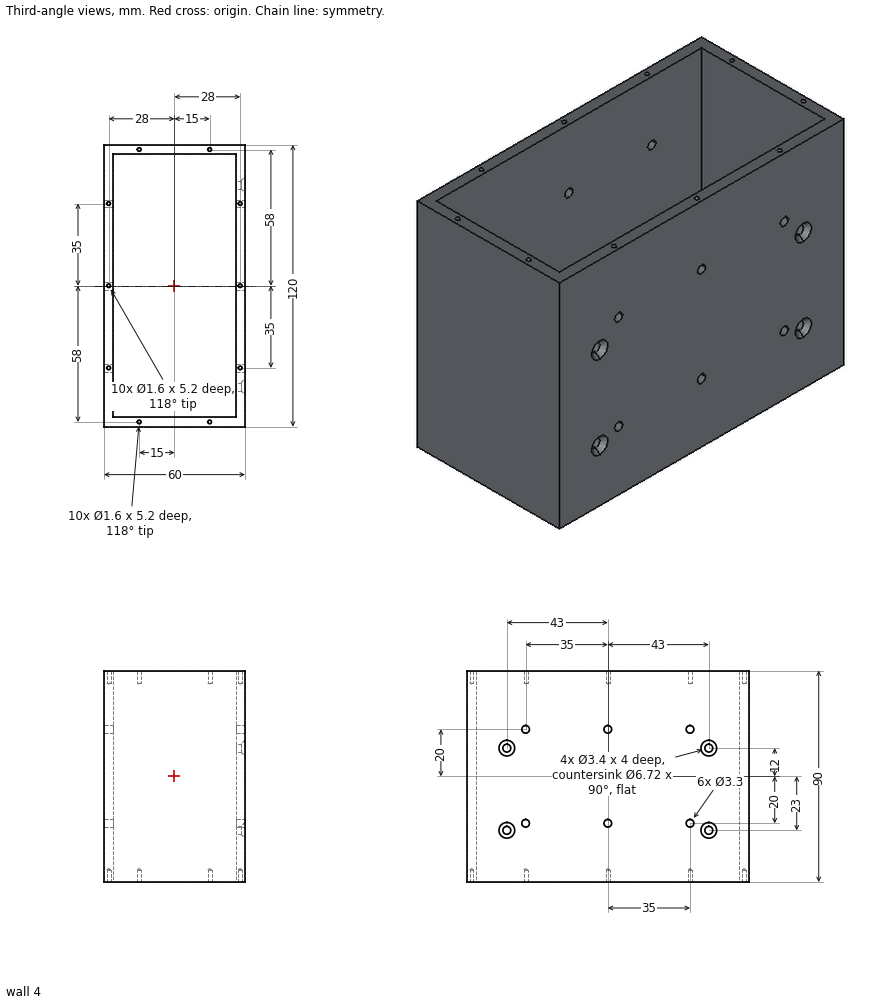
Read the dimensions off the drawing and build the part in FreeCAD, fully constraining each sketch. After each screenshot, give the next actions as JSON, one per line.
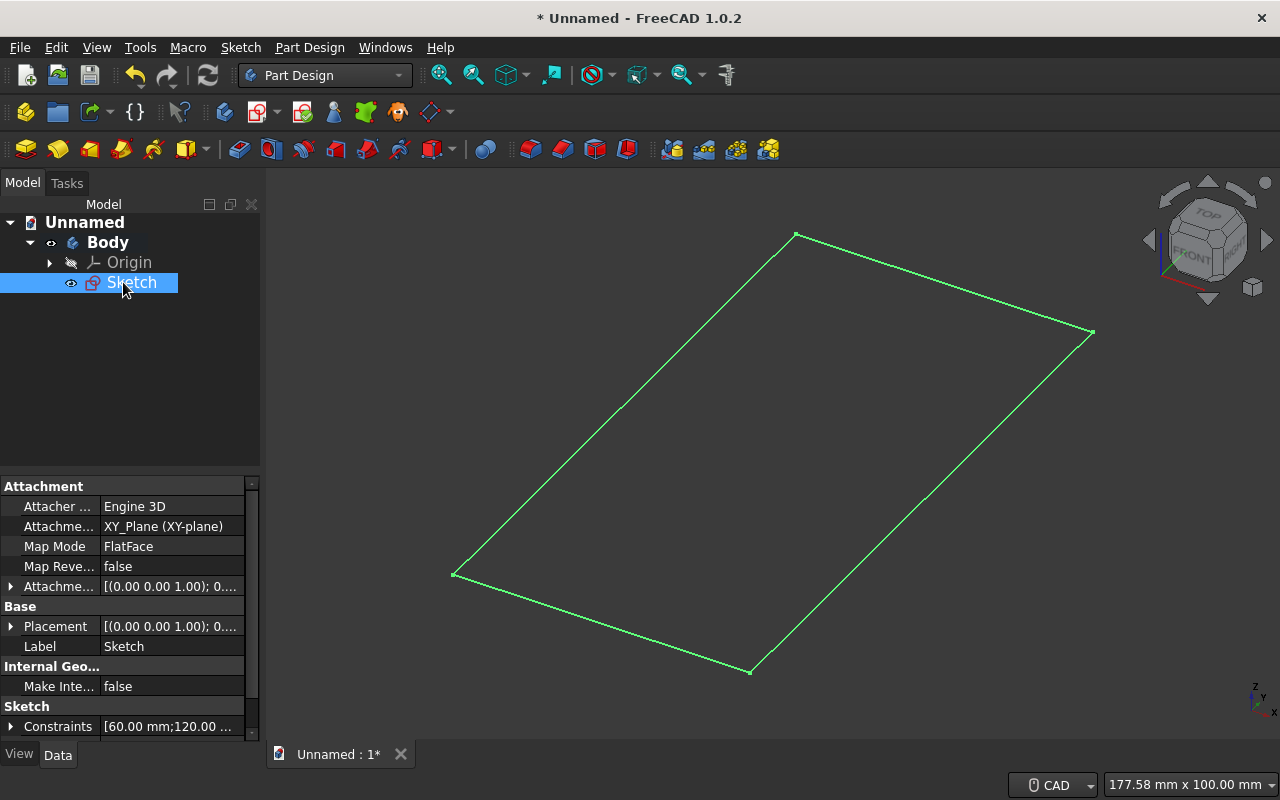
{"action": "left_click", "coordinate": [26, 150]}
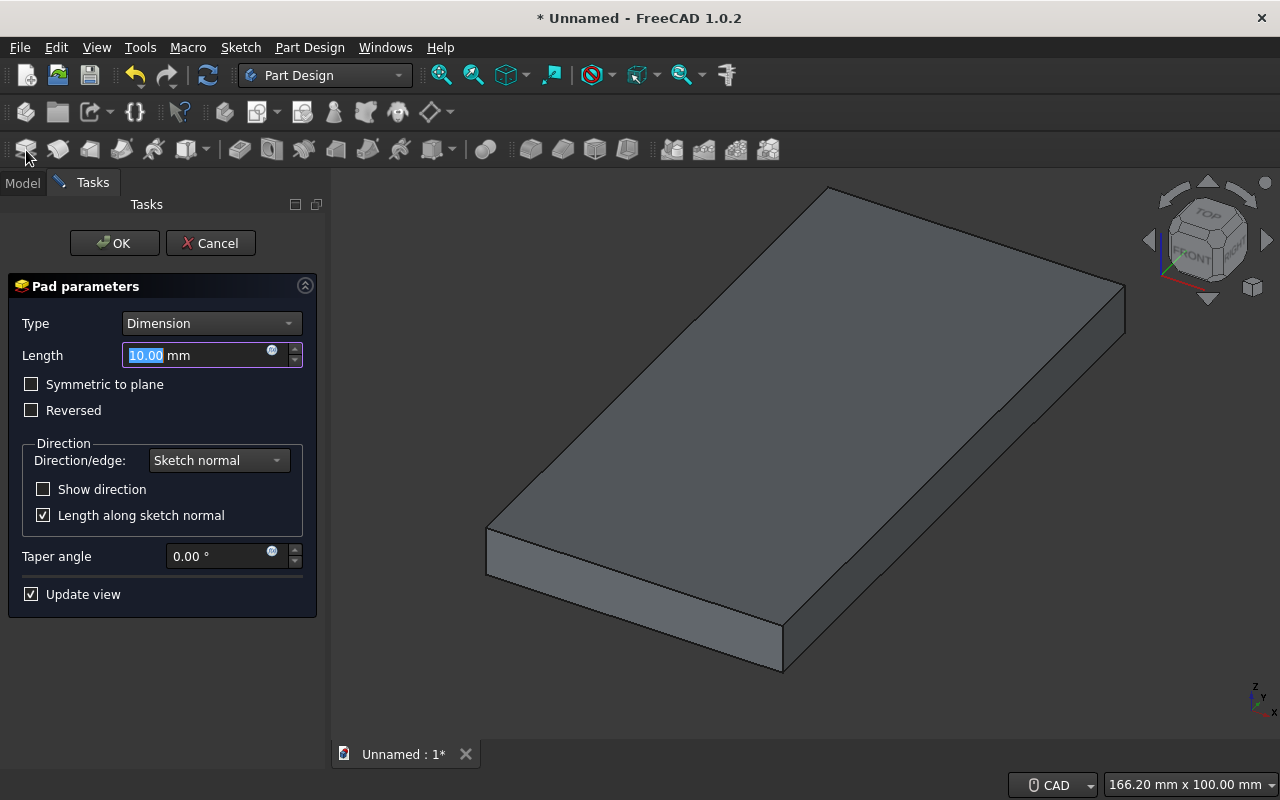
{"action": "type", "text": "90"}
{"action": "key", "text": "Tab"}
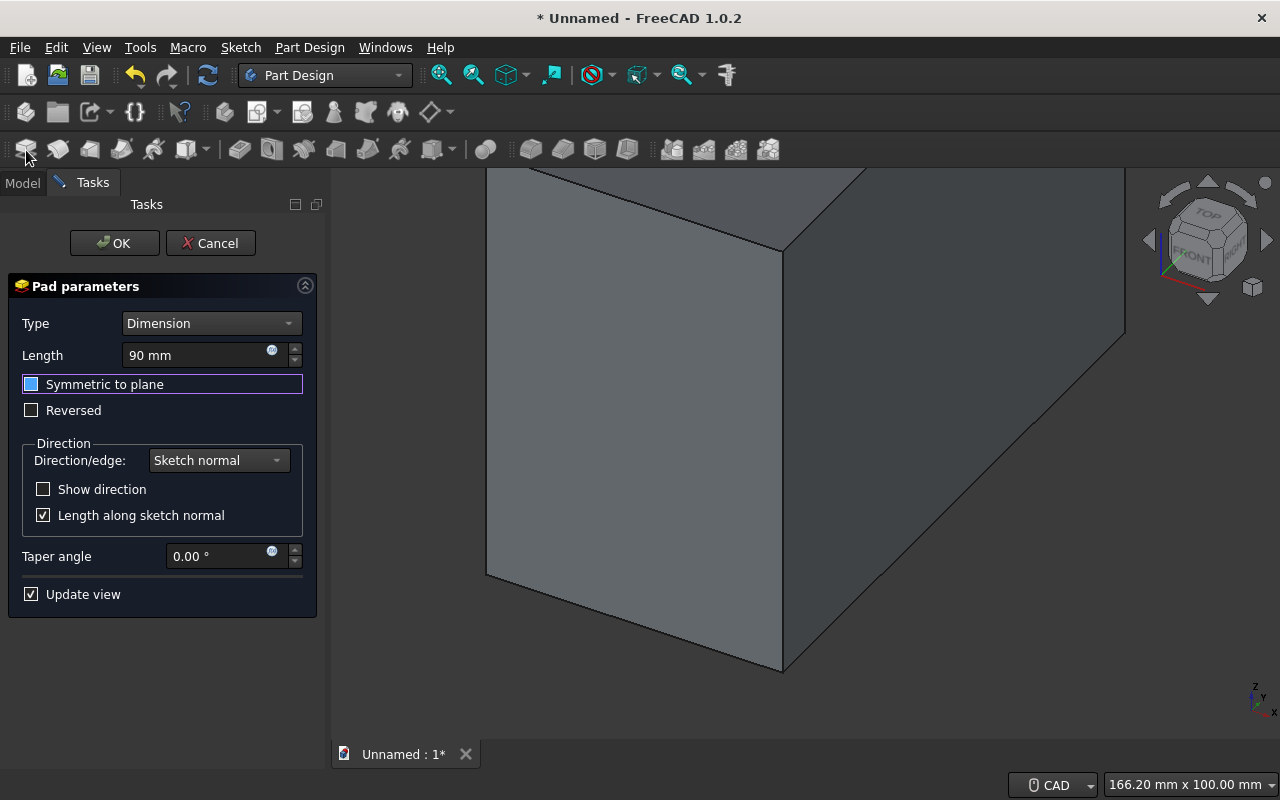
{"action": "left_click", "coordinate": [30, 384]}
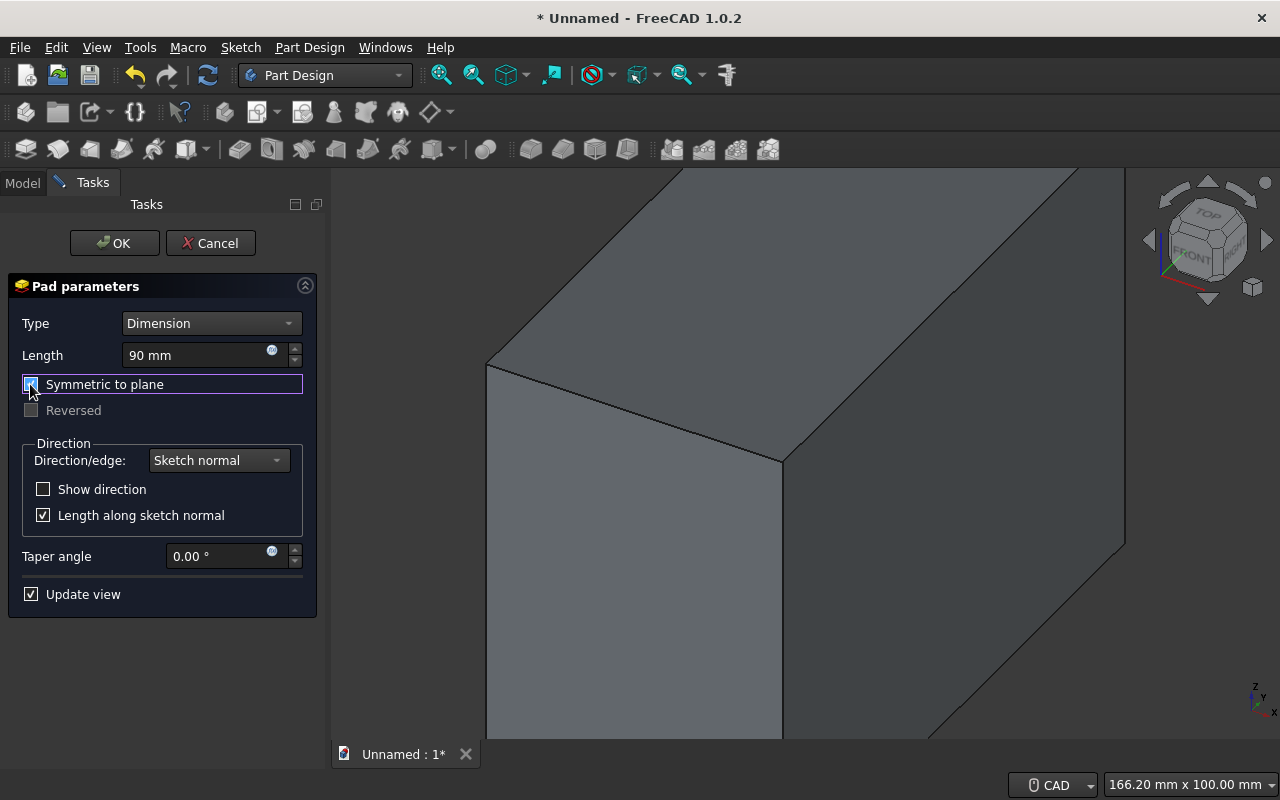
{"action": "left_click", "coordinate": [115, 243]}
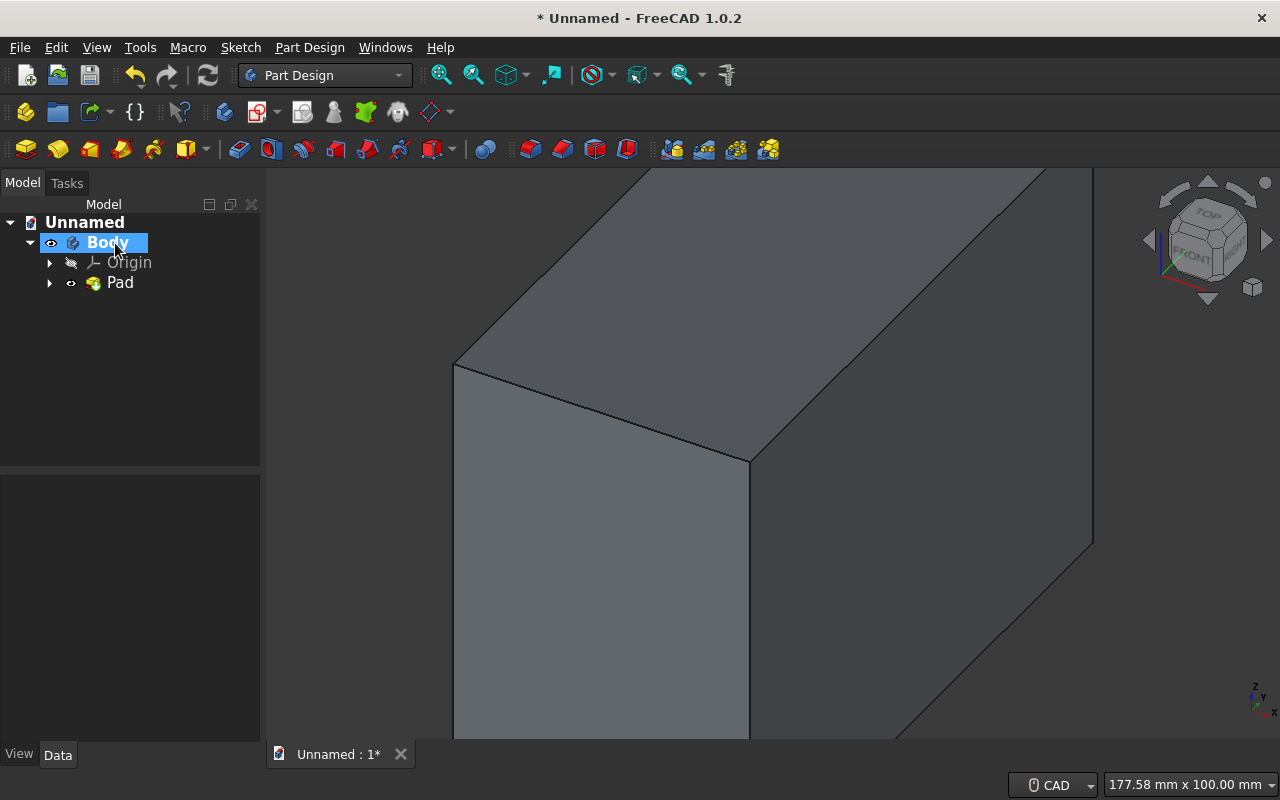
{"action": "left_click", "coordinate": [442, 76]}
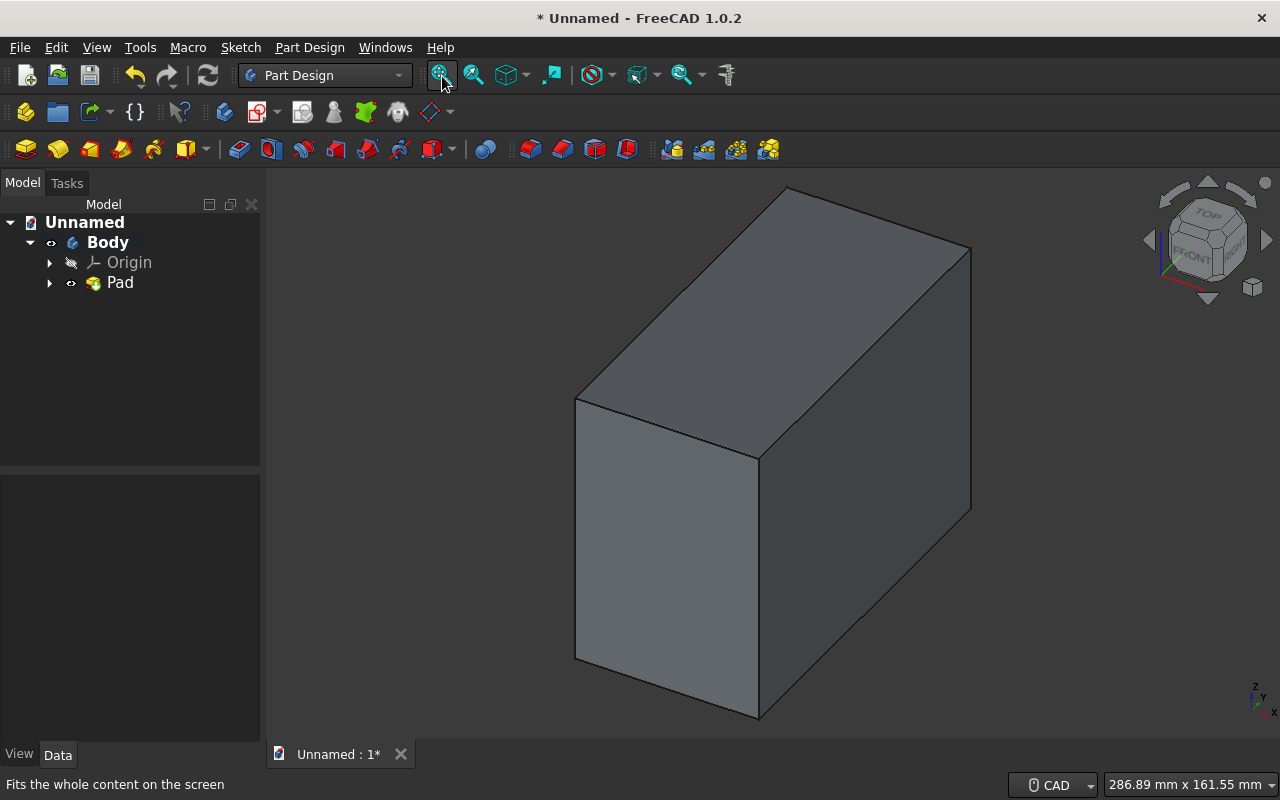
{"action": "left_click", "coordinate": [803, 292]}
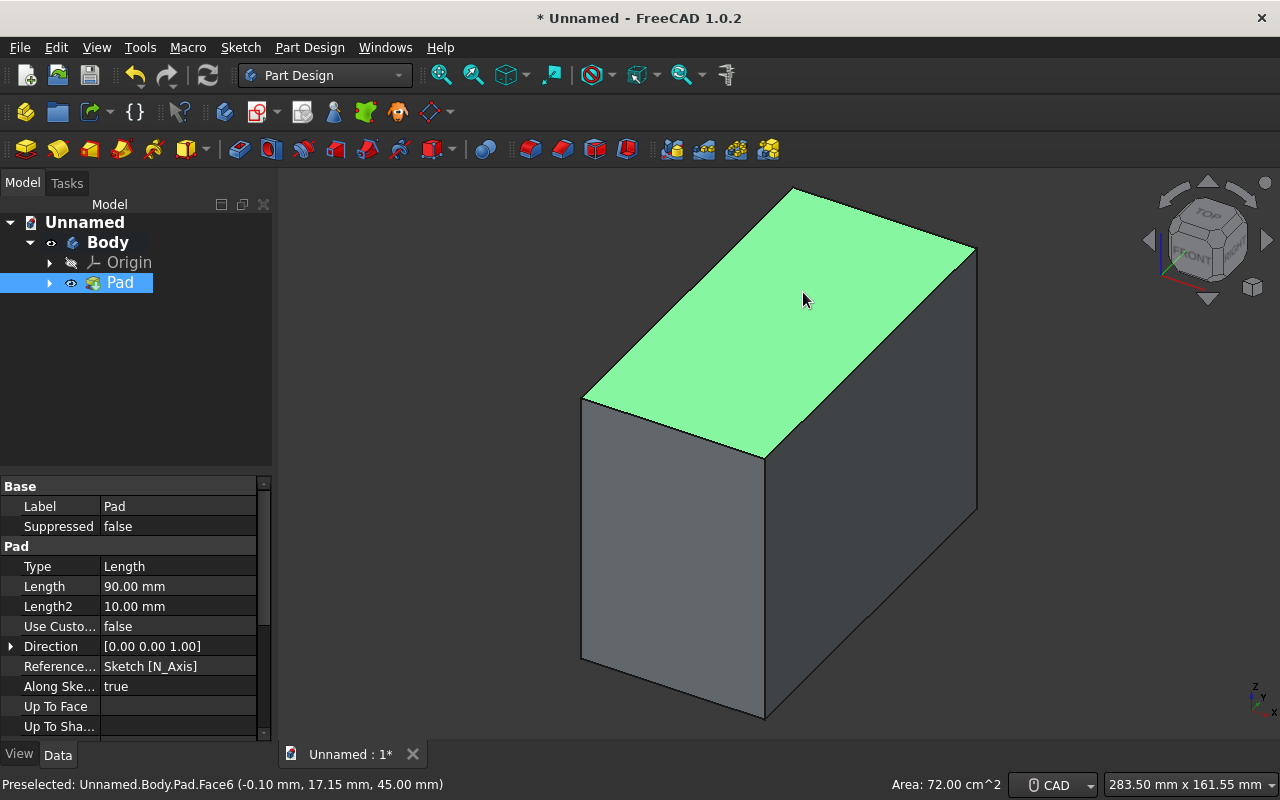
{"action": "key", "text": "0"}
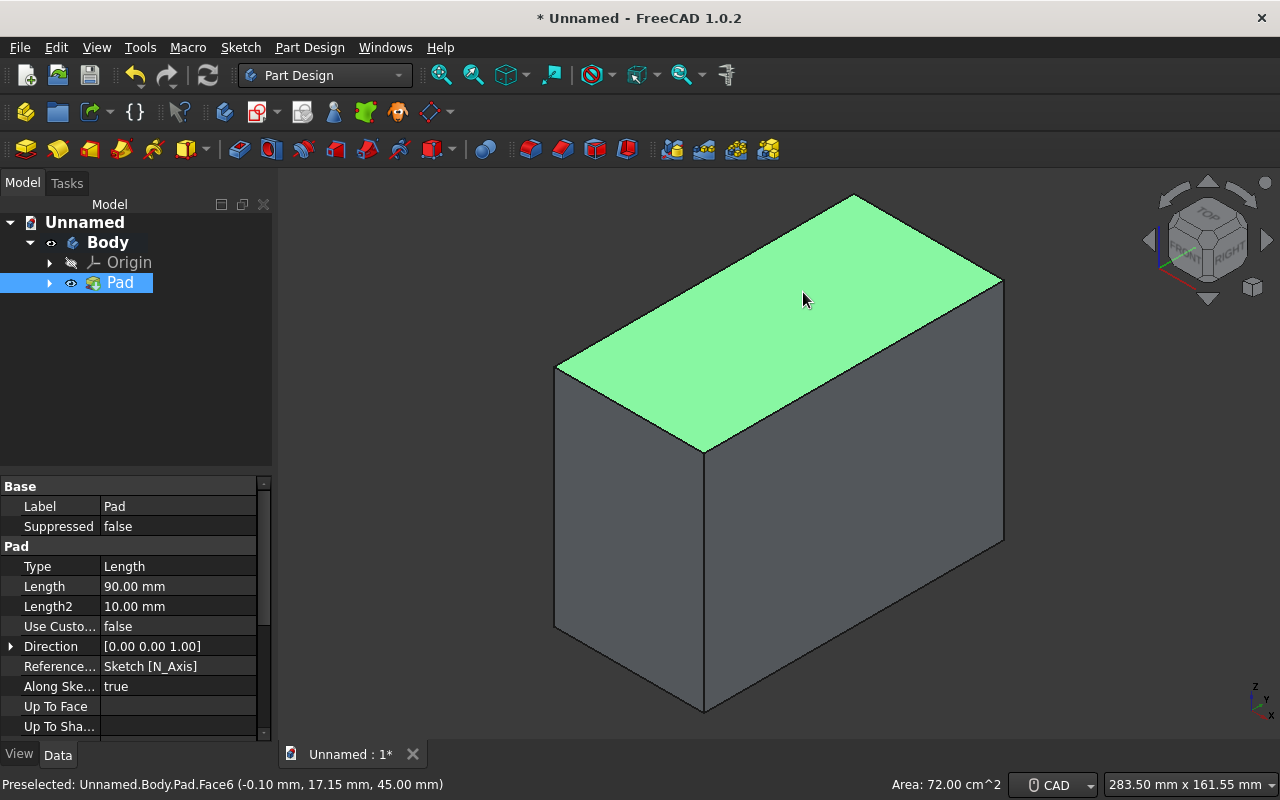
{"action": "key", "text": "2"}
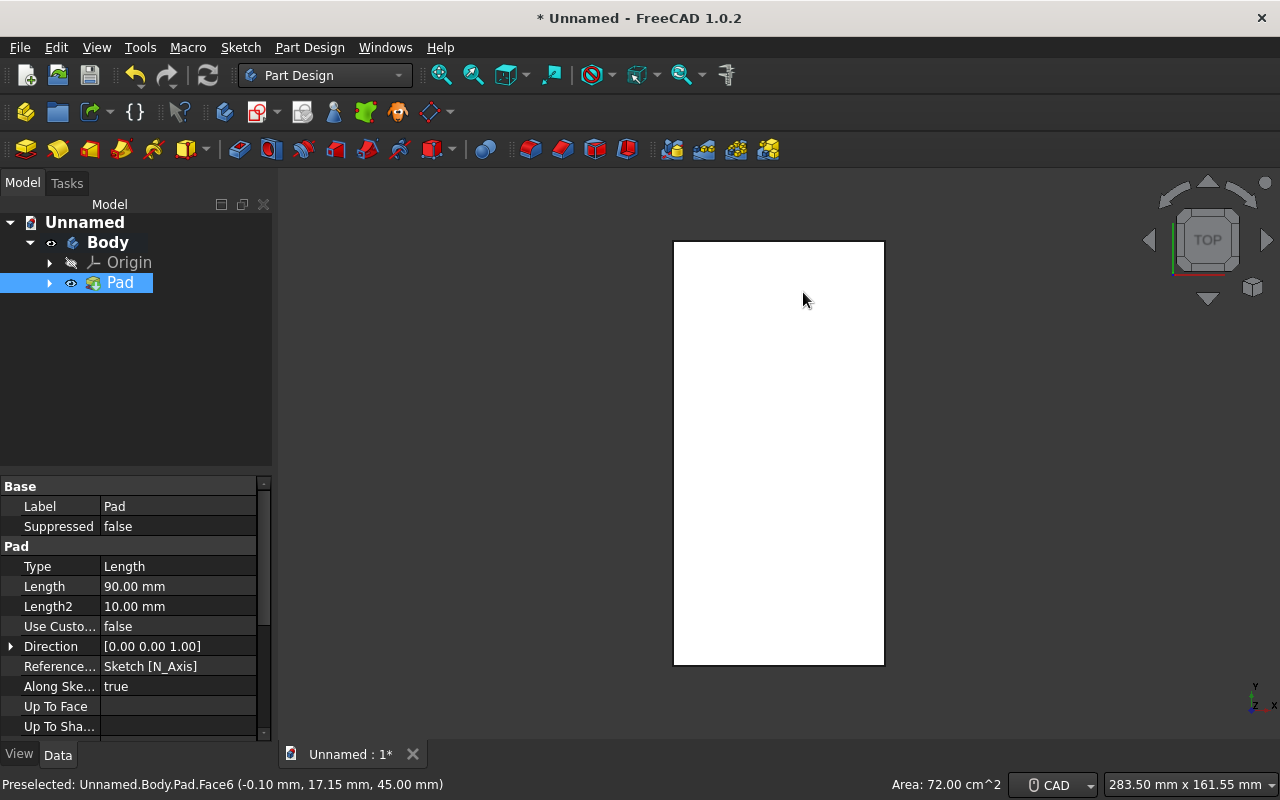
{"action": "key", "text": "1"}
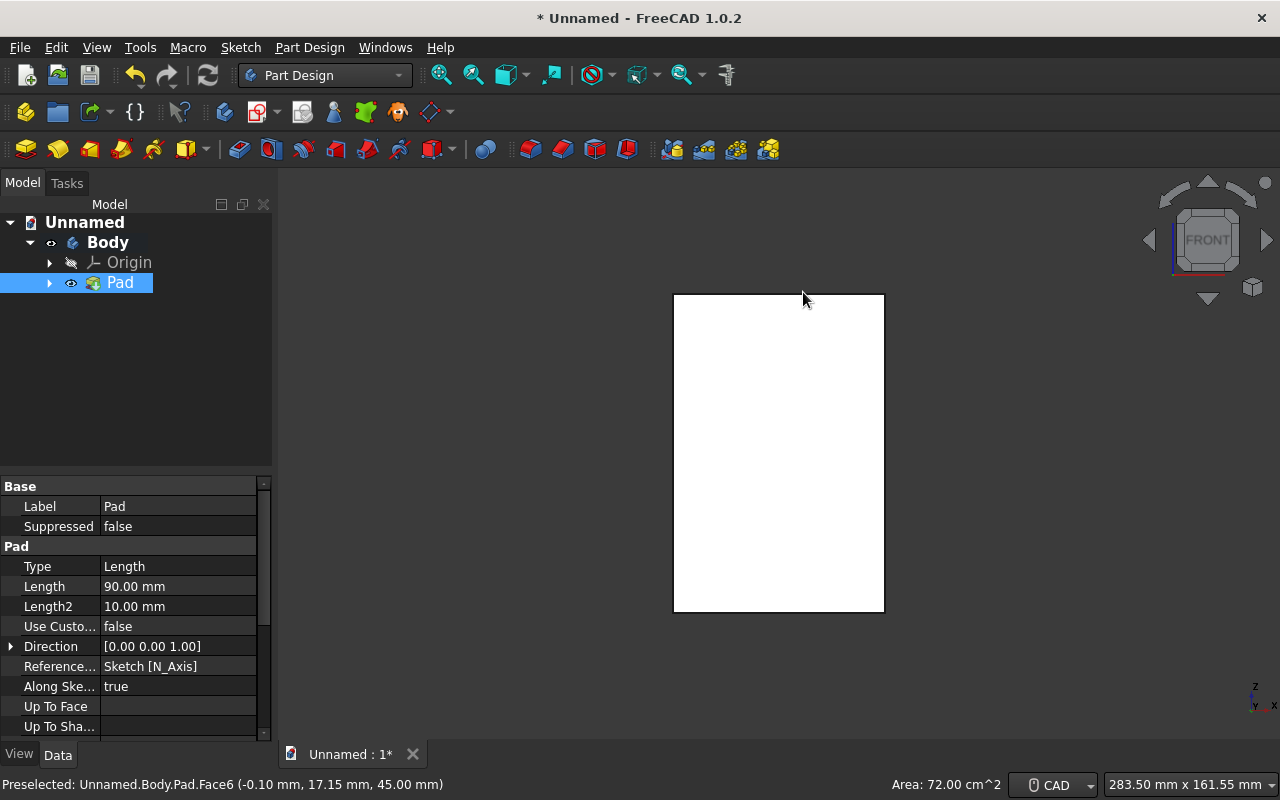
{"action": "key", "text": "3"}